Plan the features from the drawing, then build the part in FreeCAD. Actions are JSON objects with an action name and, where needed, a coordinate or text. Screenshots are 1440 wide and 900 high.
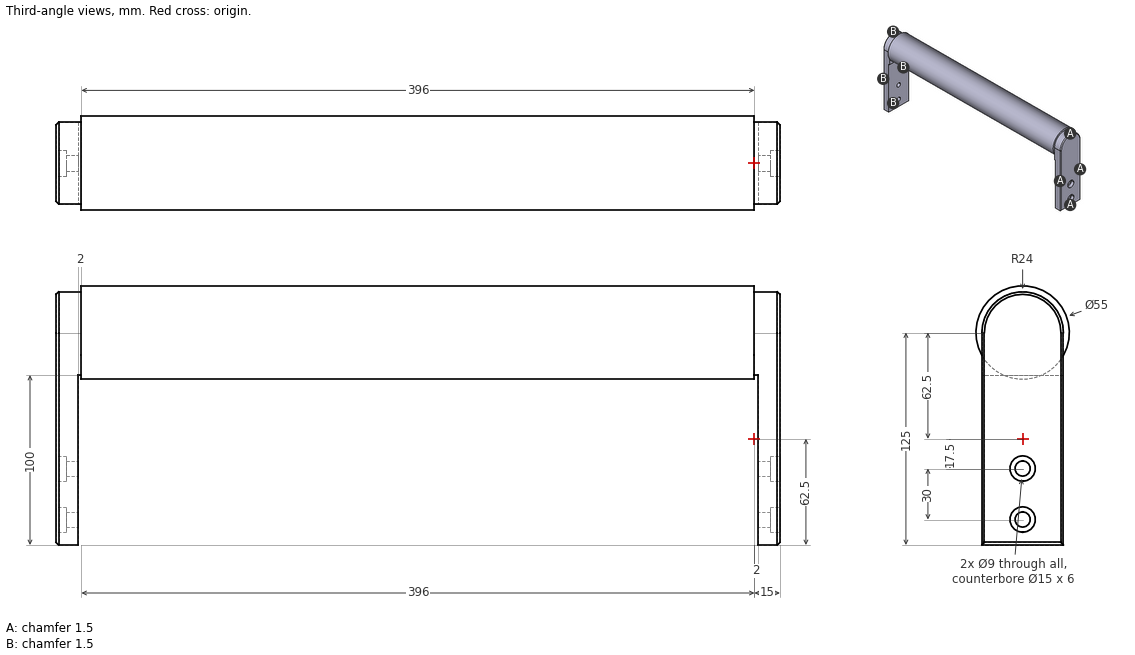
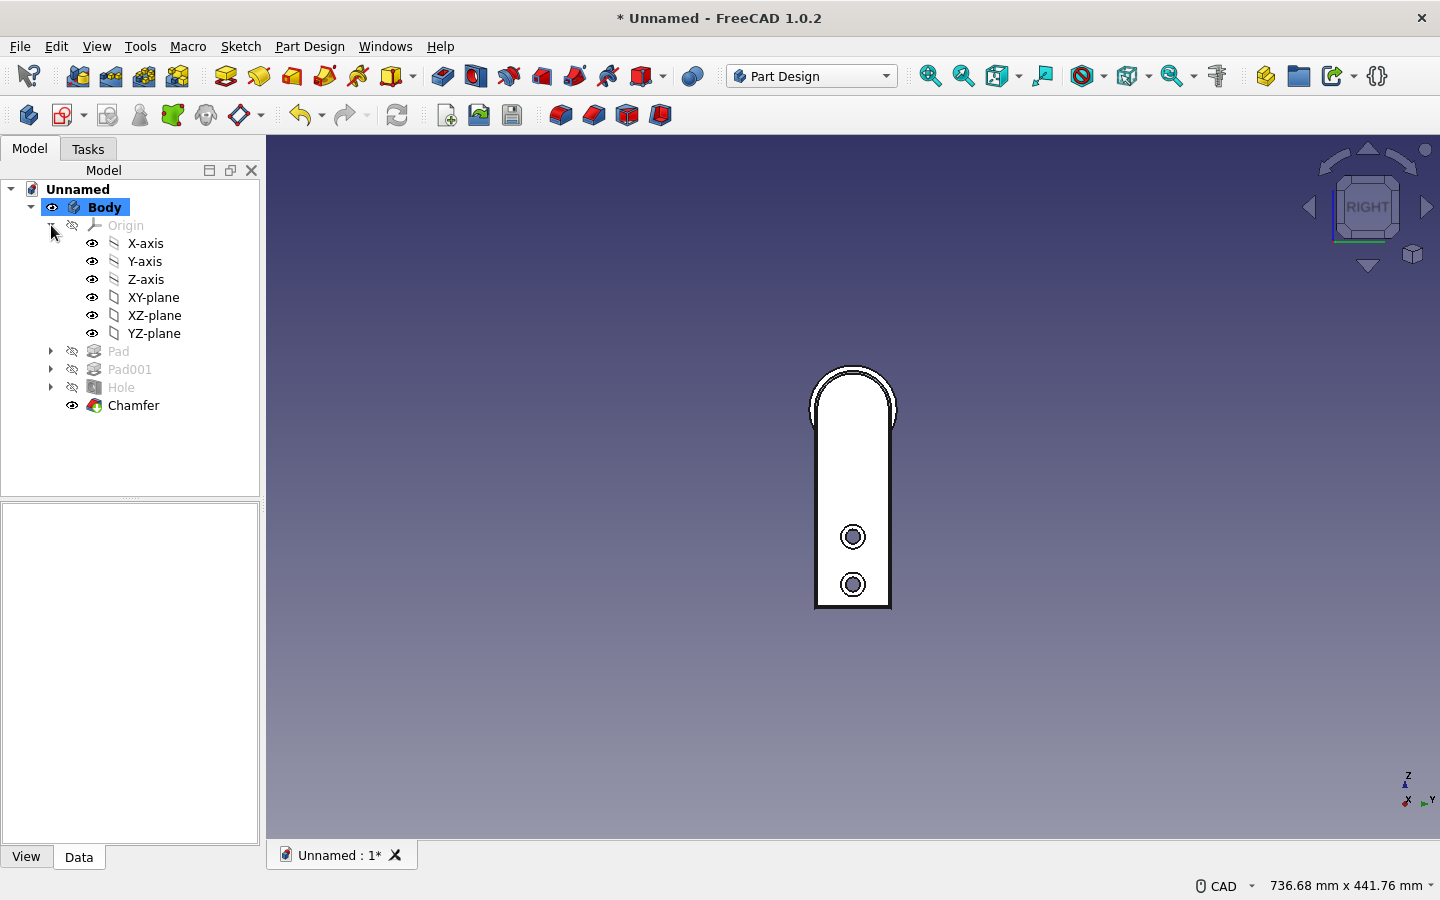
{"action": "left_click", "coordinate": [137, 333]}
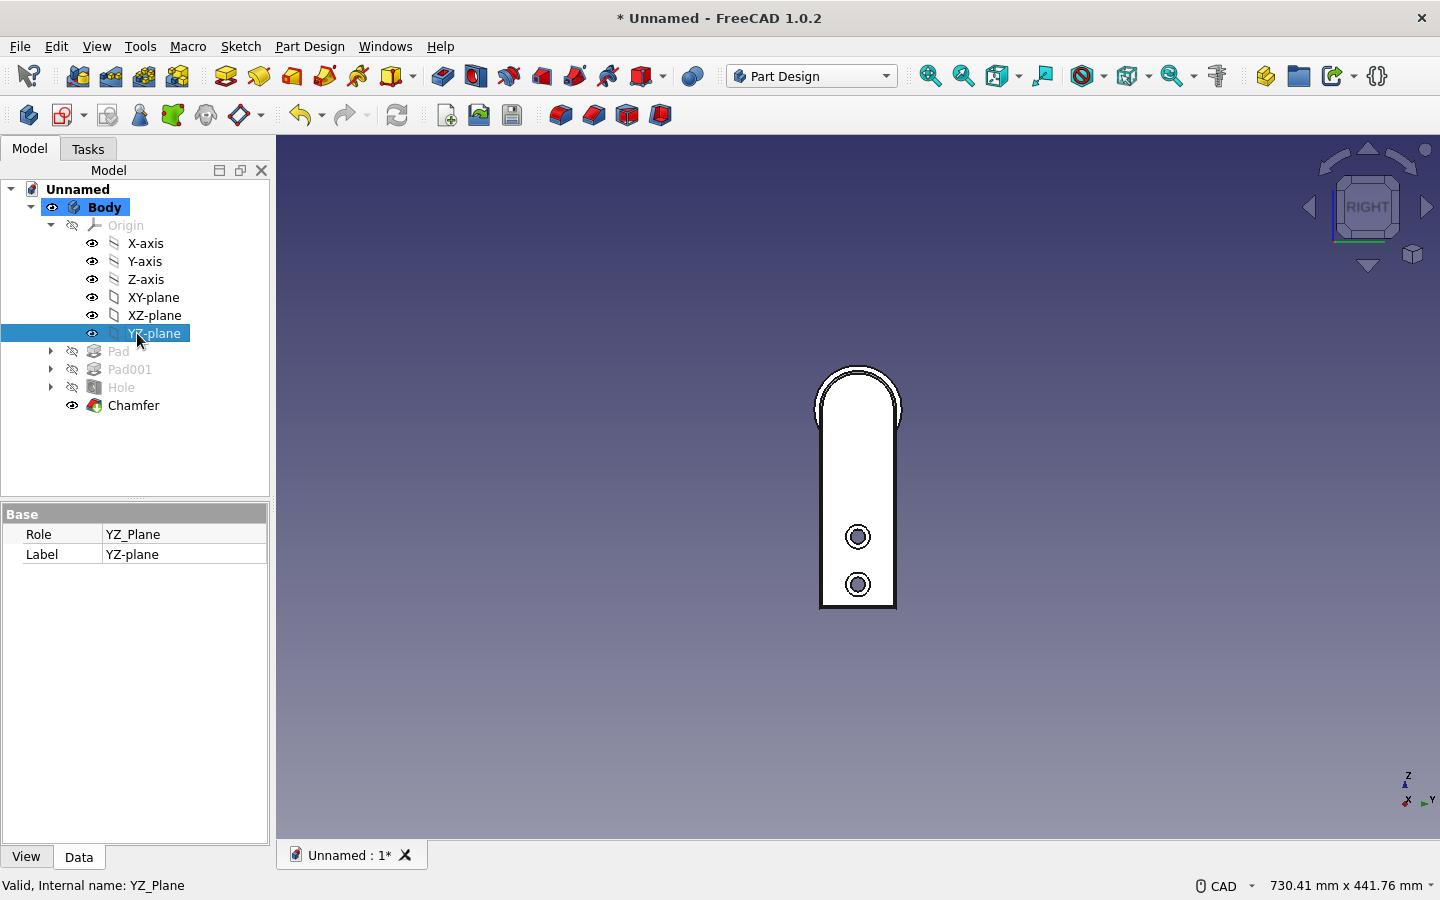
{"action": "left_click", "coordinate": [238, 116]}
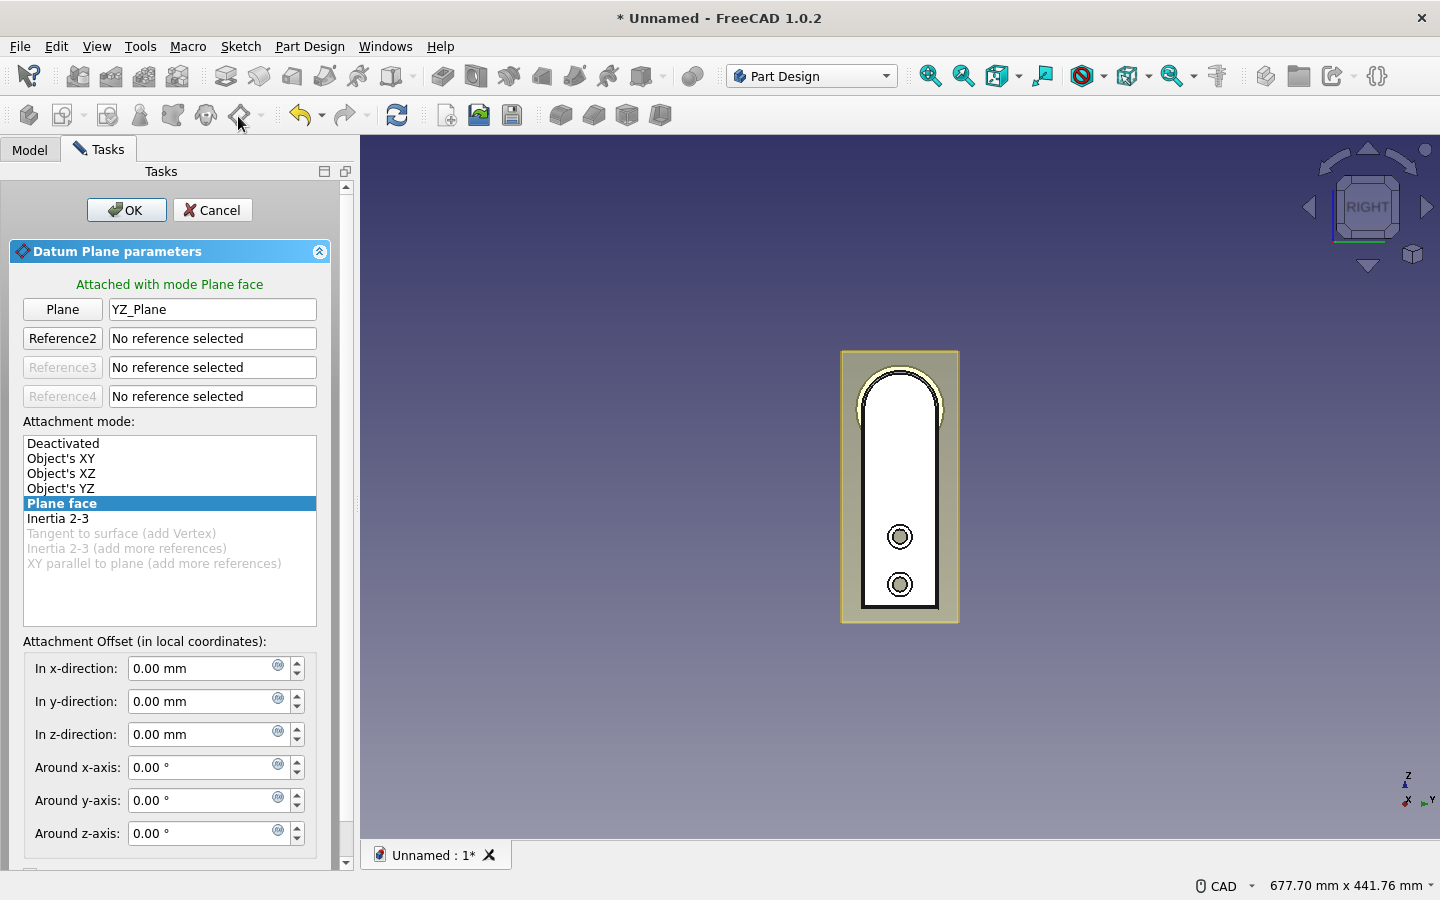
{"action": "triple_click", "coordinate": [210, 734]}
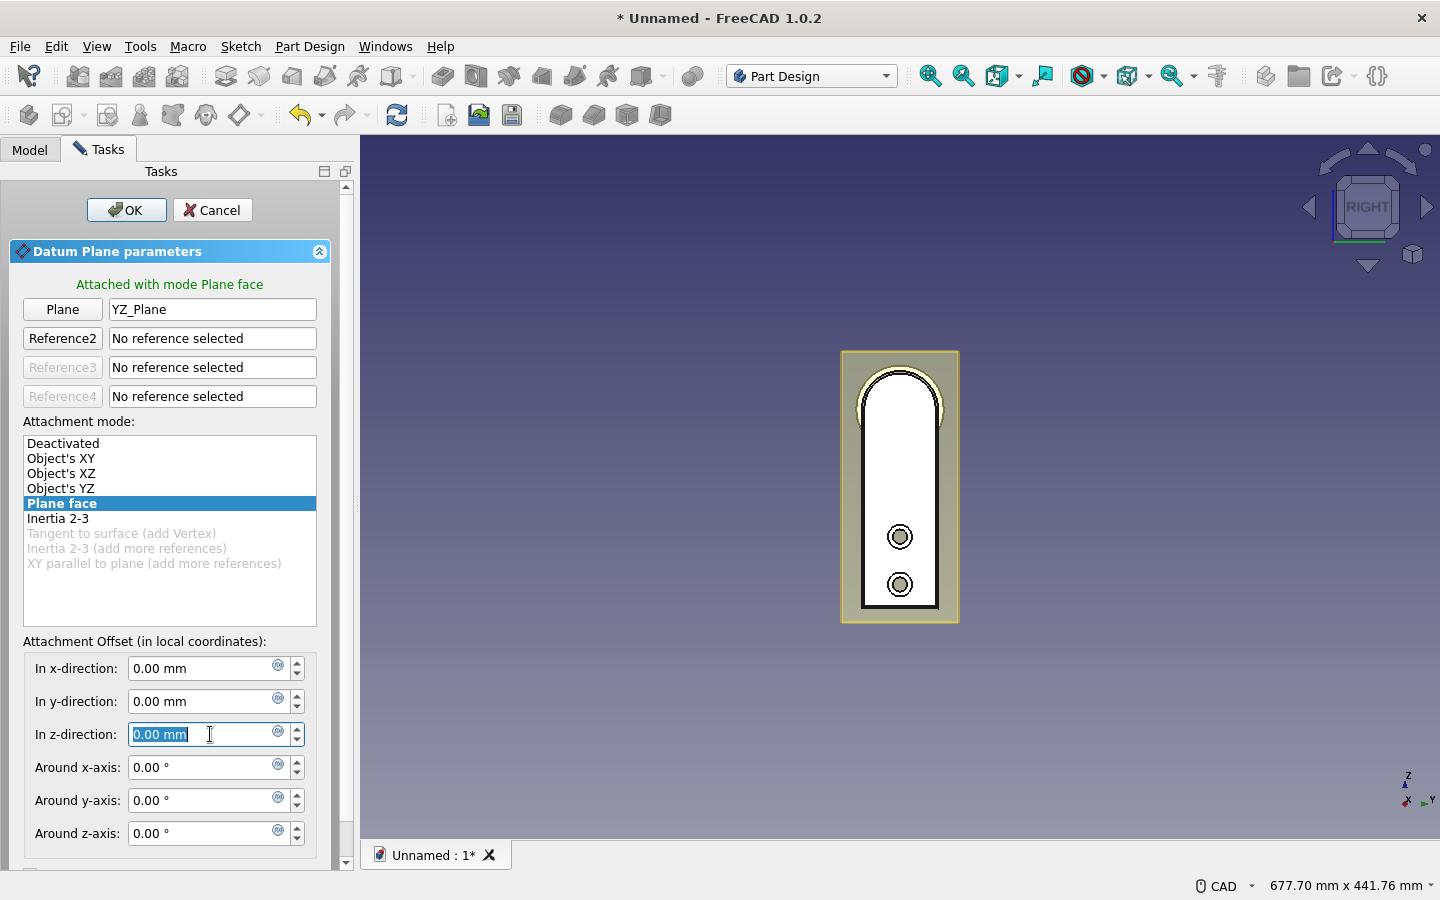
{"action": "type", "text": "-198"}
{"action": "key", "text": "Tab"}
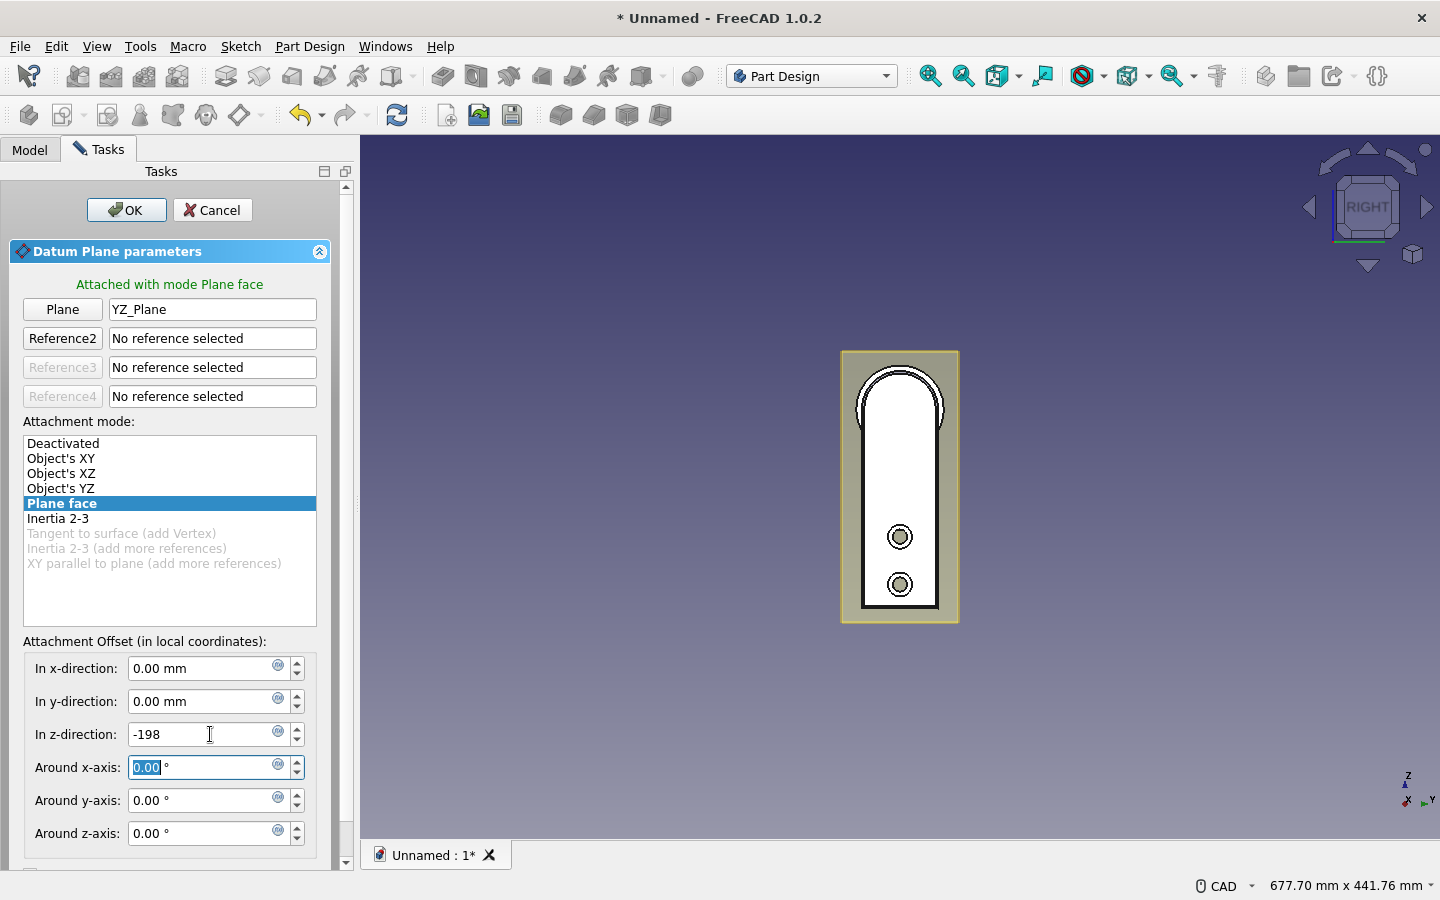
{"action": "left_click", "coordinate": [127, 210]}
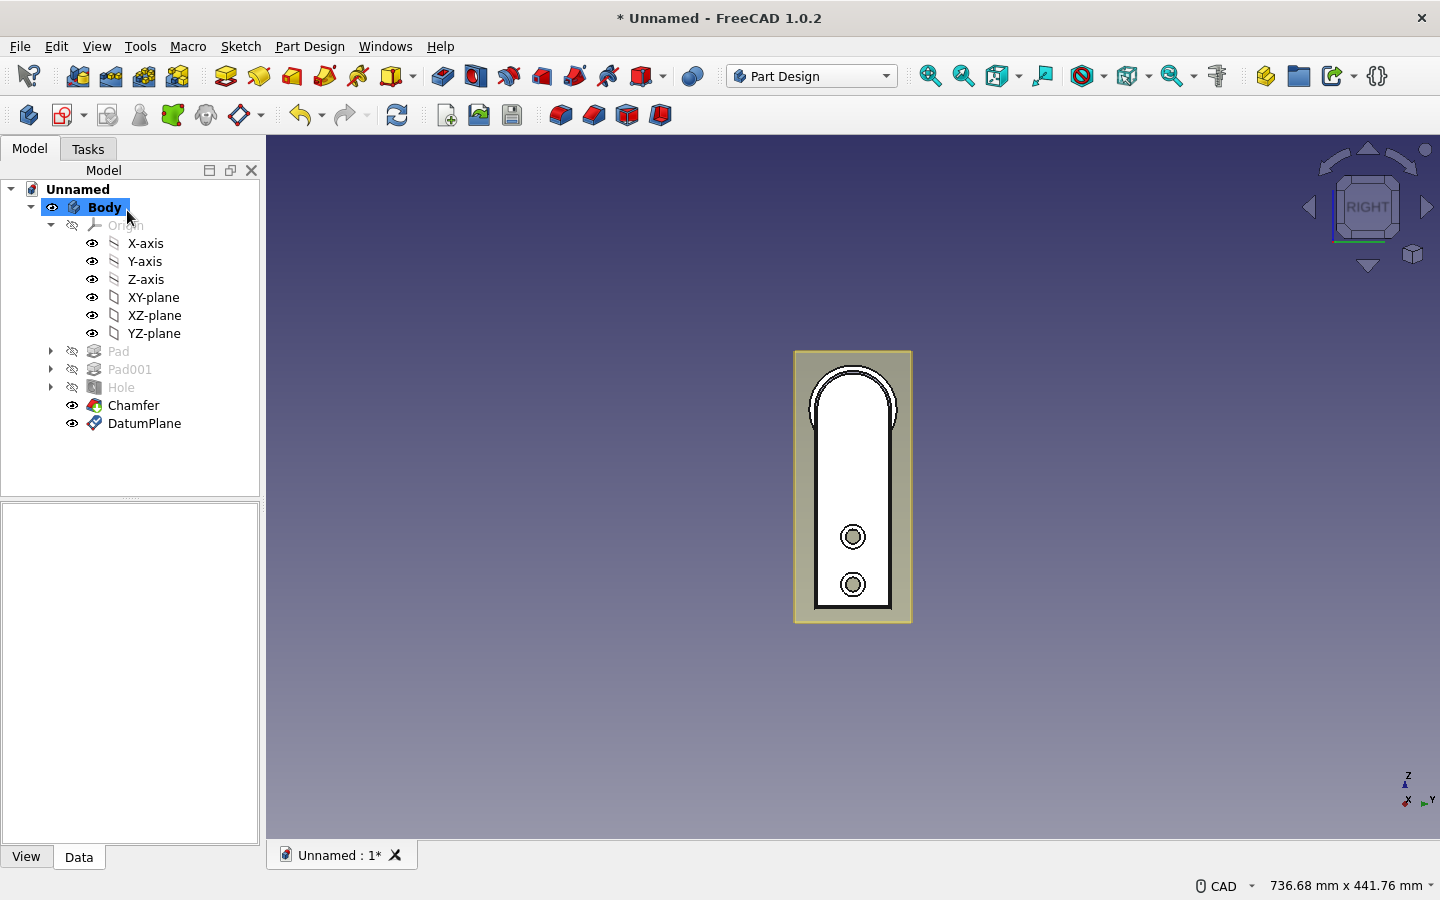
{"action": "left_click", "coordinate": [117, 351]}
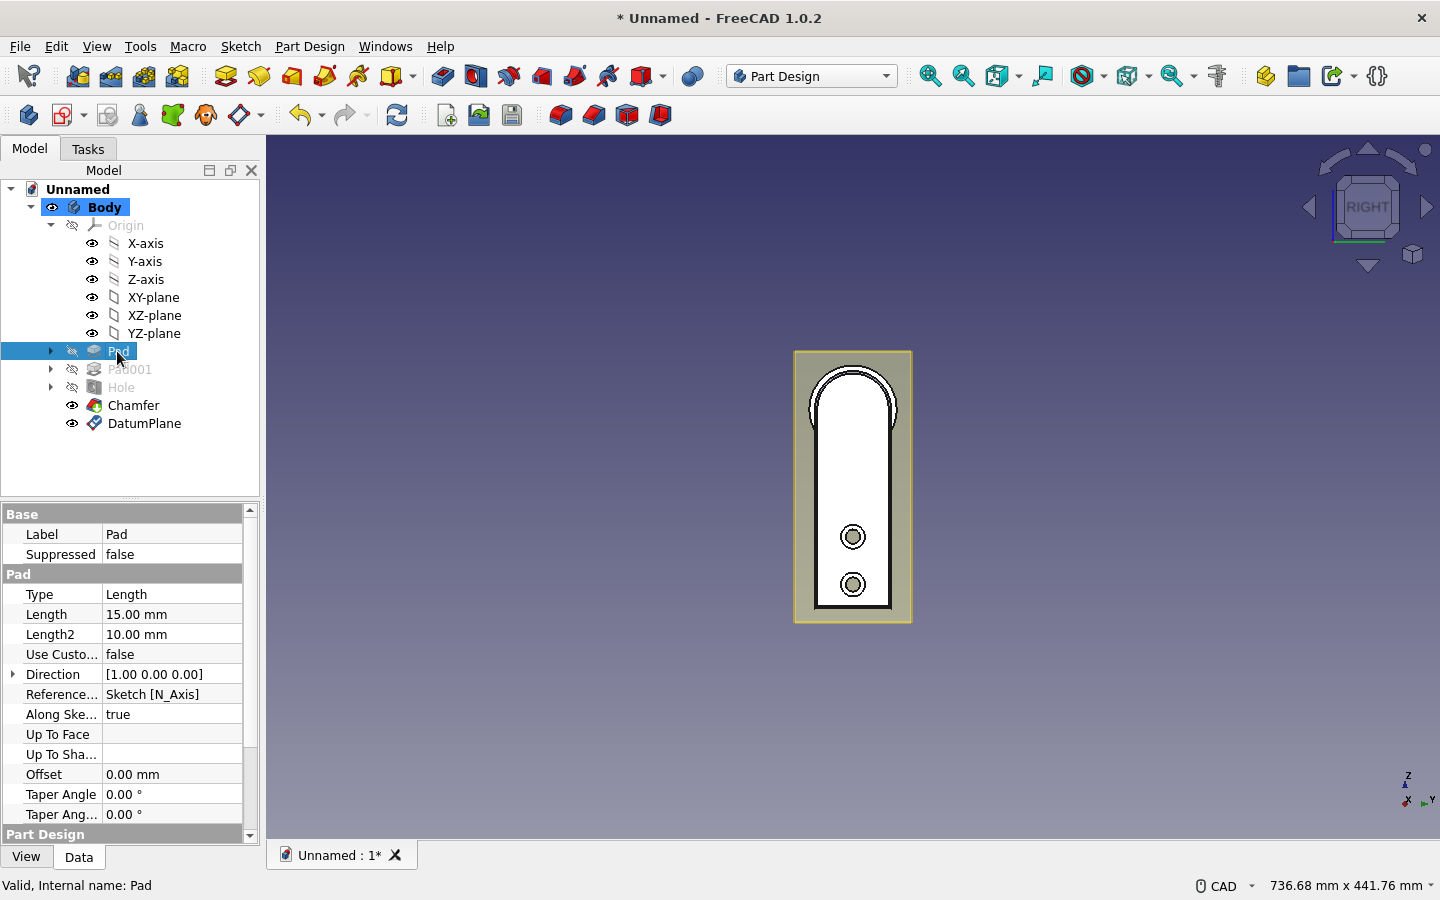
{"action": "left_click", "coordinate": [117, 387], "text": "ctrl"}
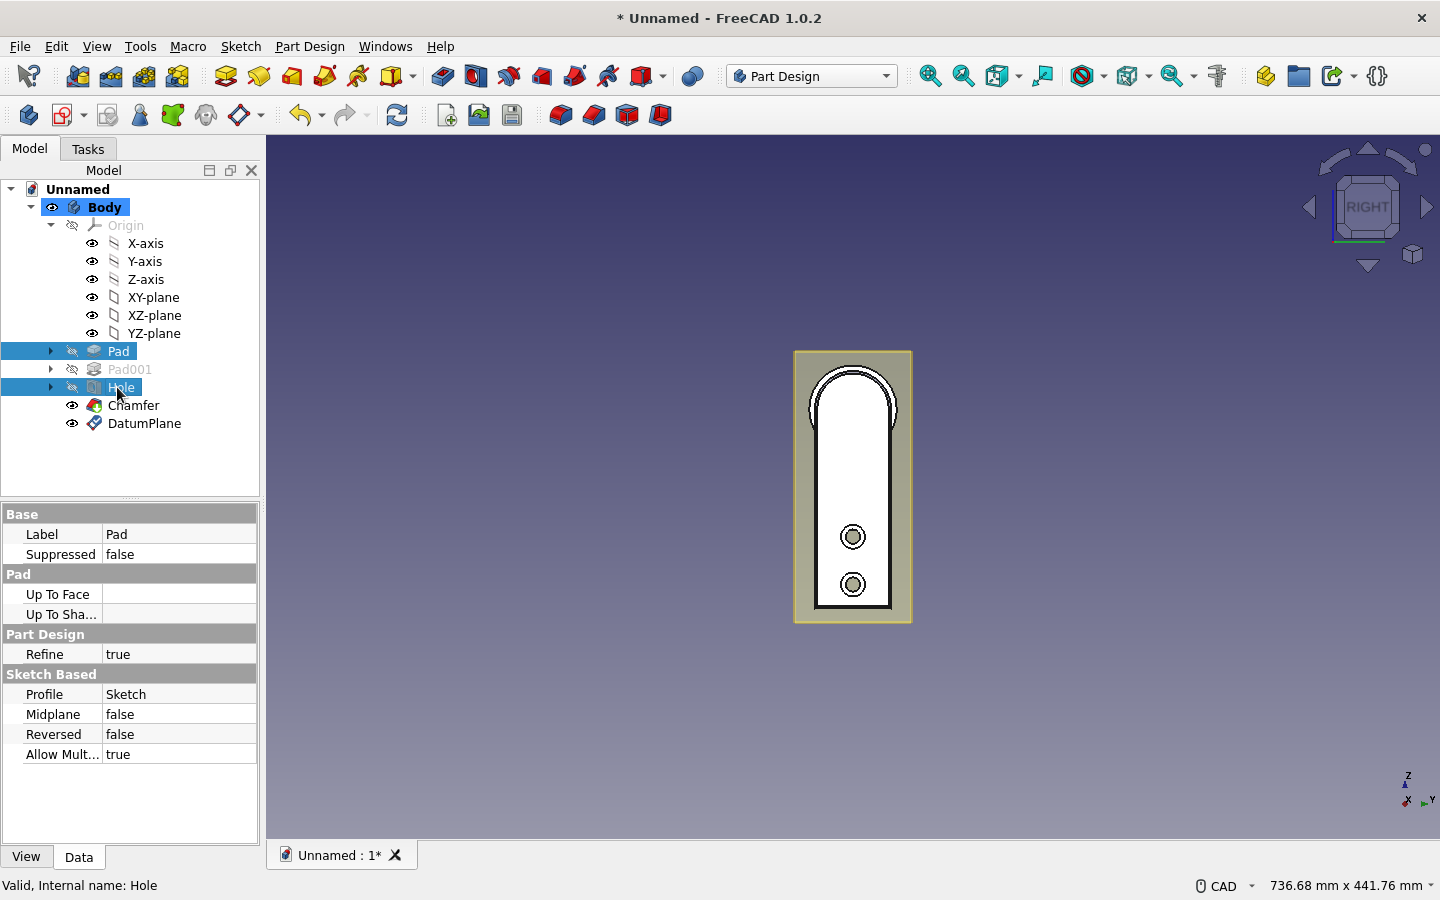
{"action": "left_click", "coordinate": [78, 76]}